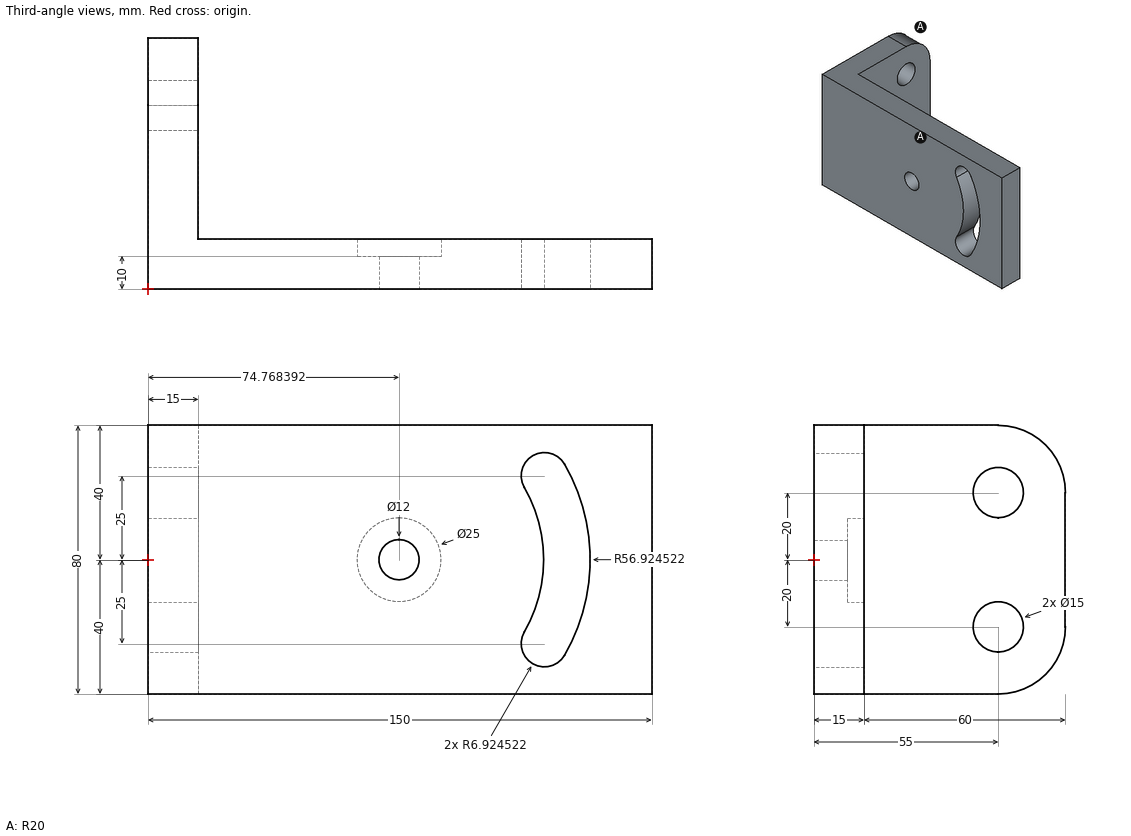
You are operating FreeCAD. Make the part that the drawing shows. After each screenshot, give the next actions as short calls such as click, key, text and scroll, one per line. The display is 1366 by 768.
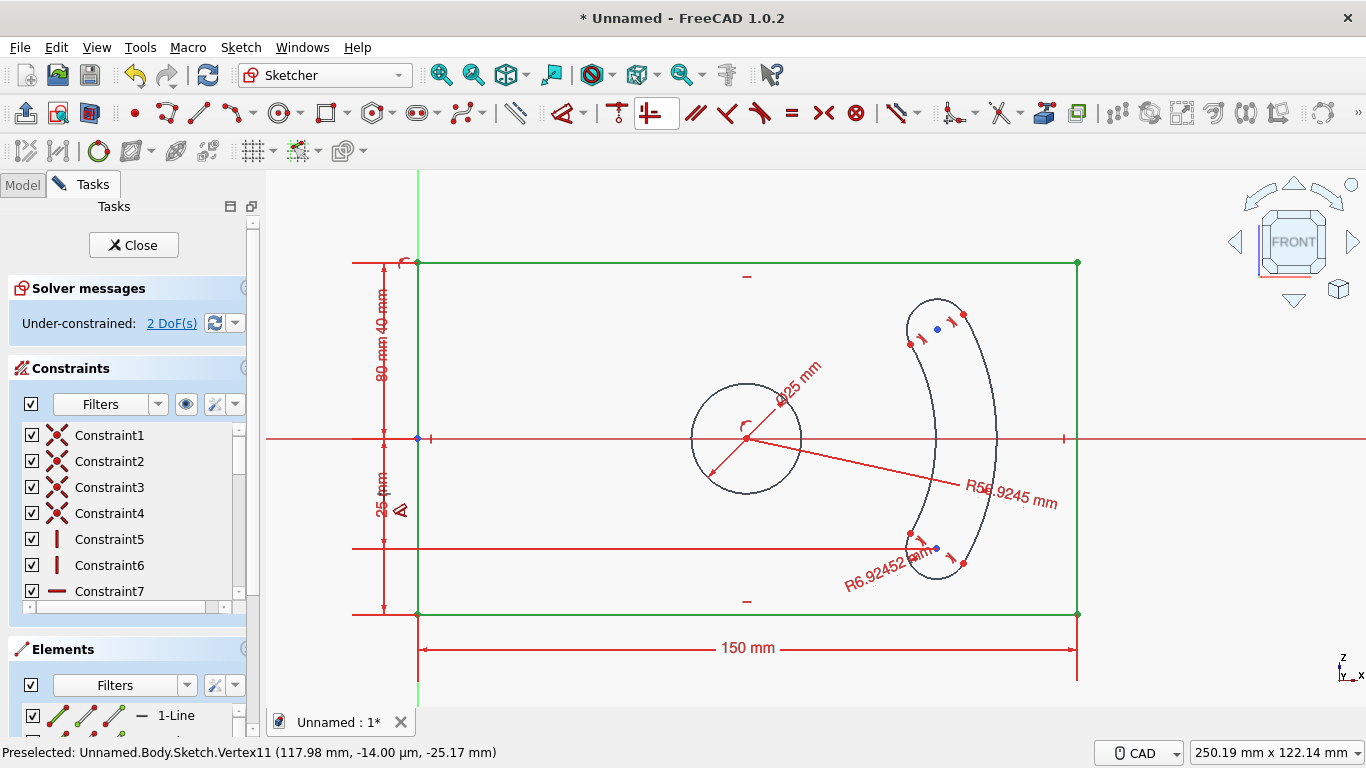
click(937, 330)
click(384, 384)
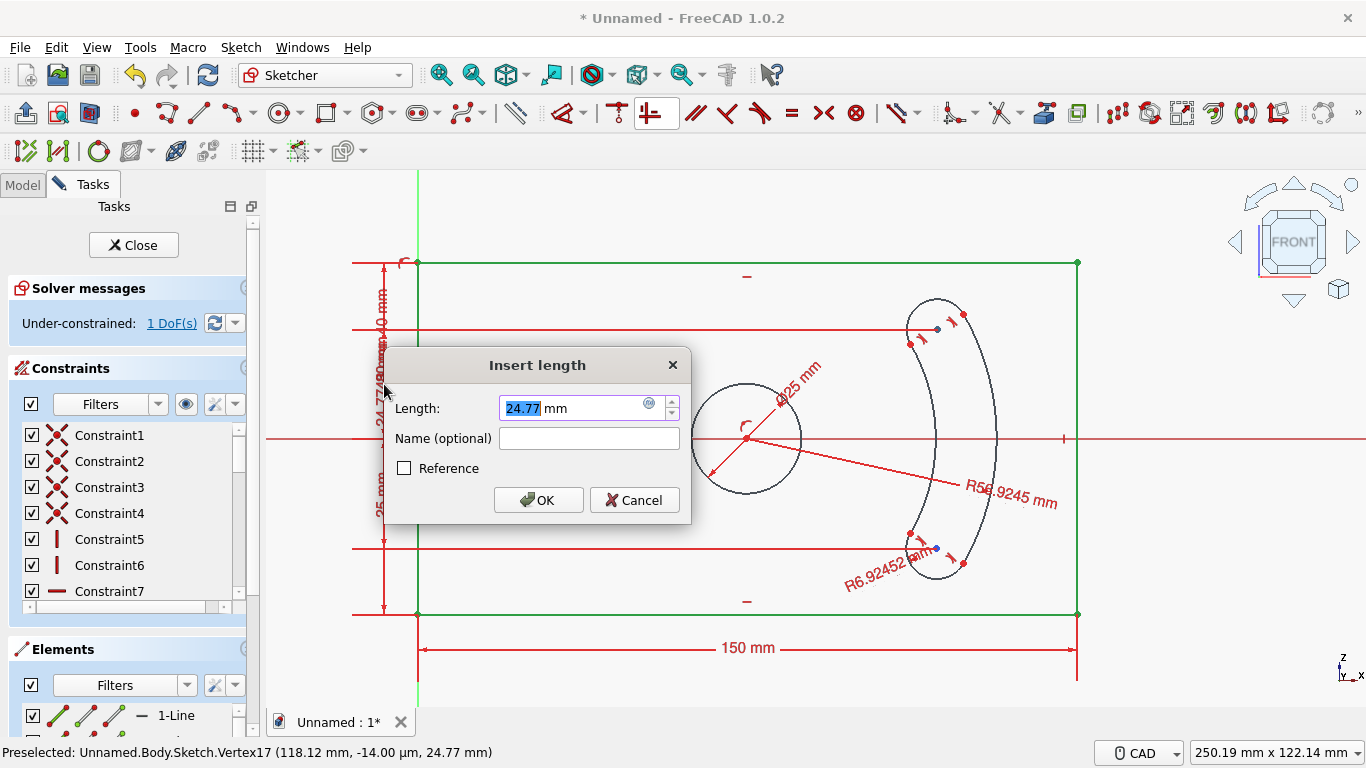
text(25)
key(Return)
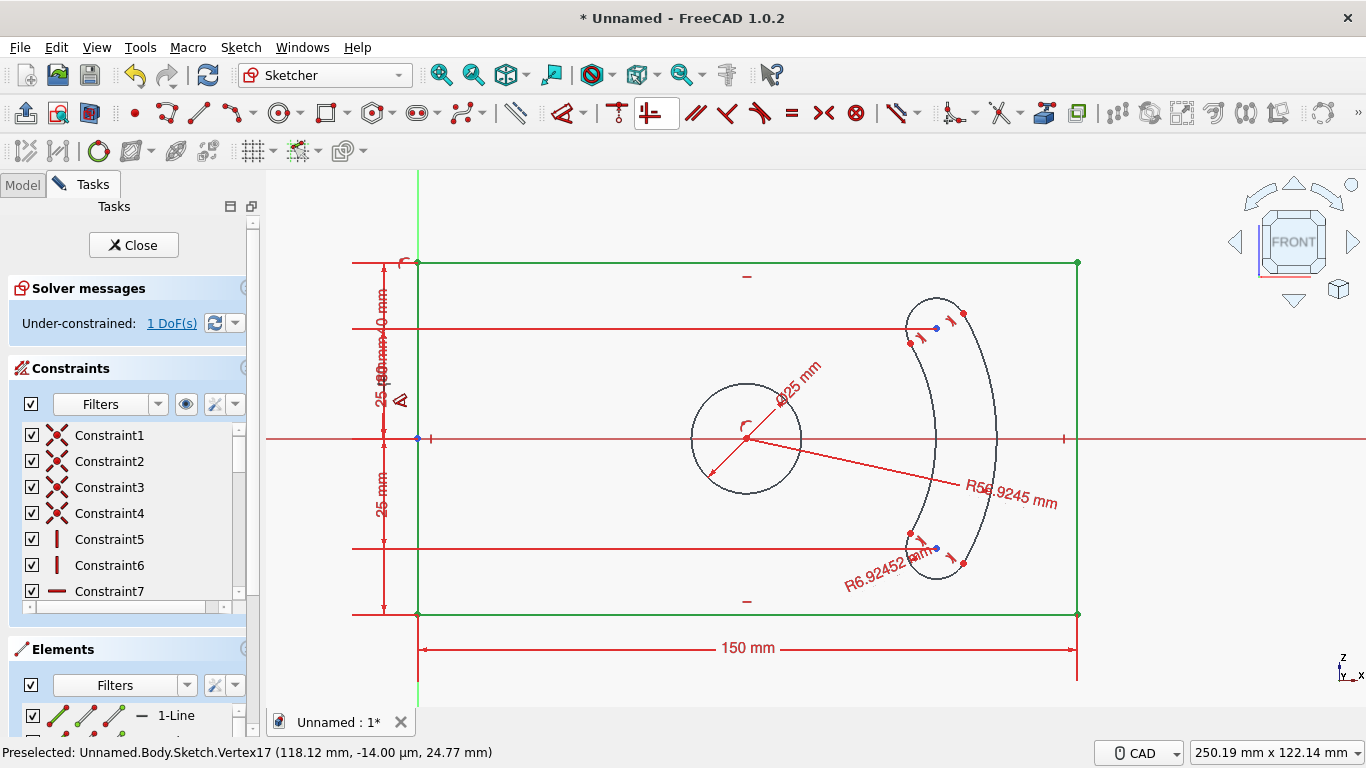
click(746, 439)
click(582, 473)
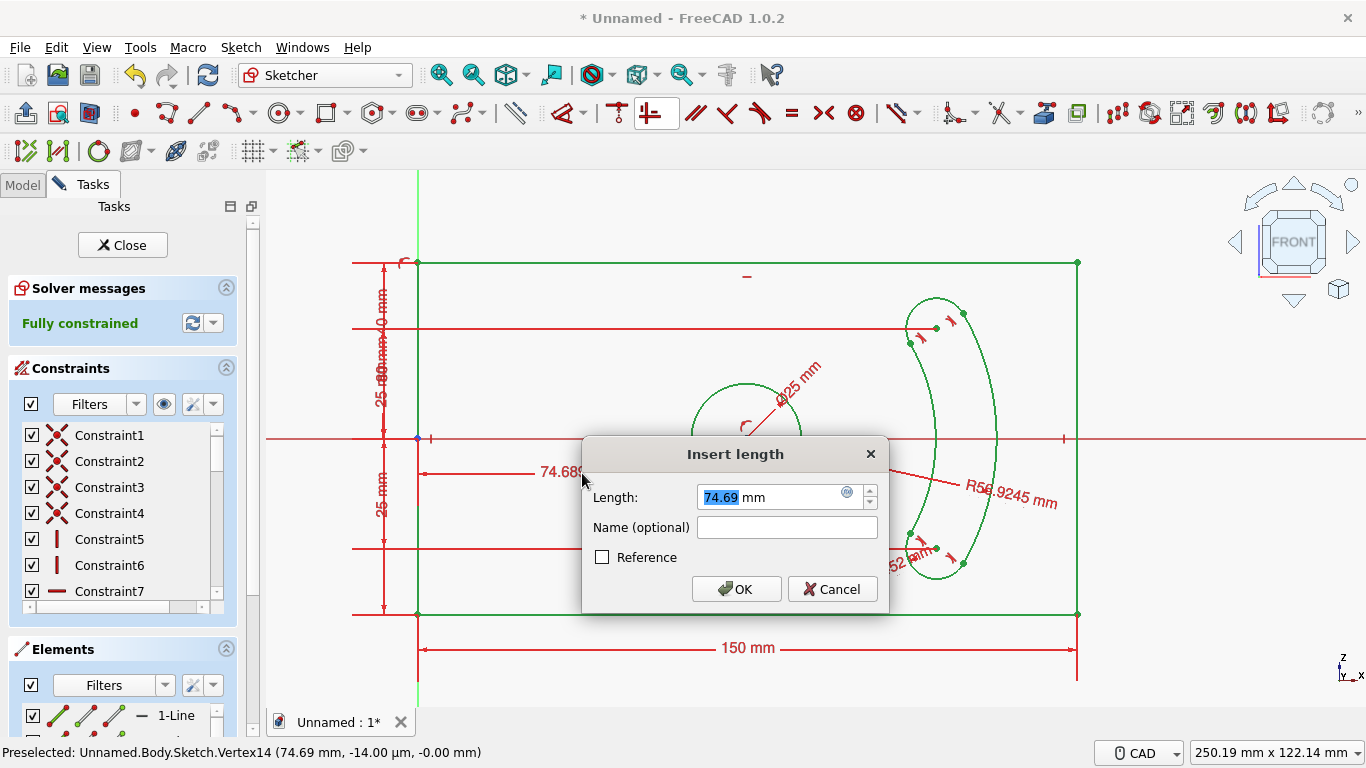
text(74.768392)
key(Return)
key(Escape)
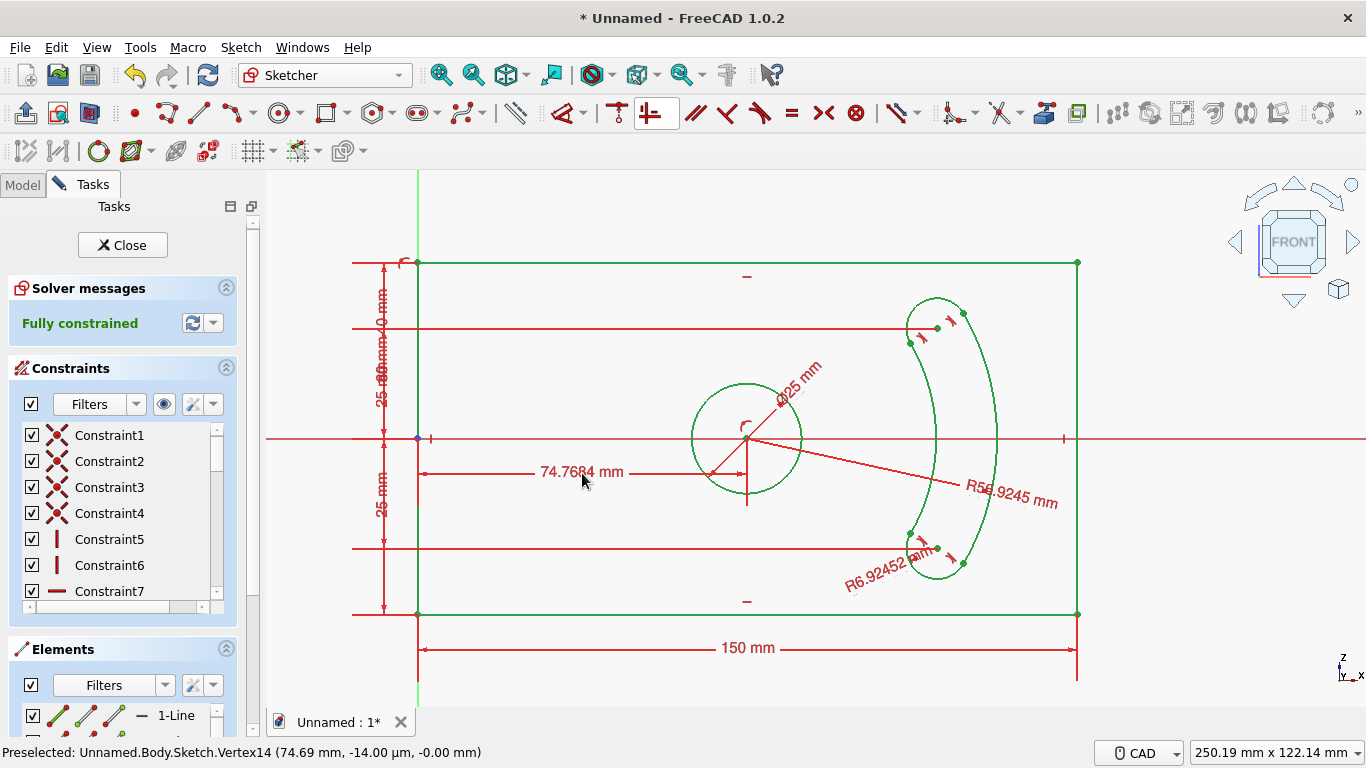
click(123, 245)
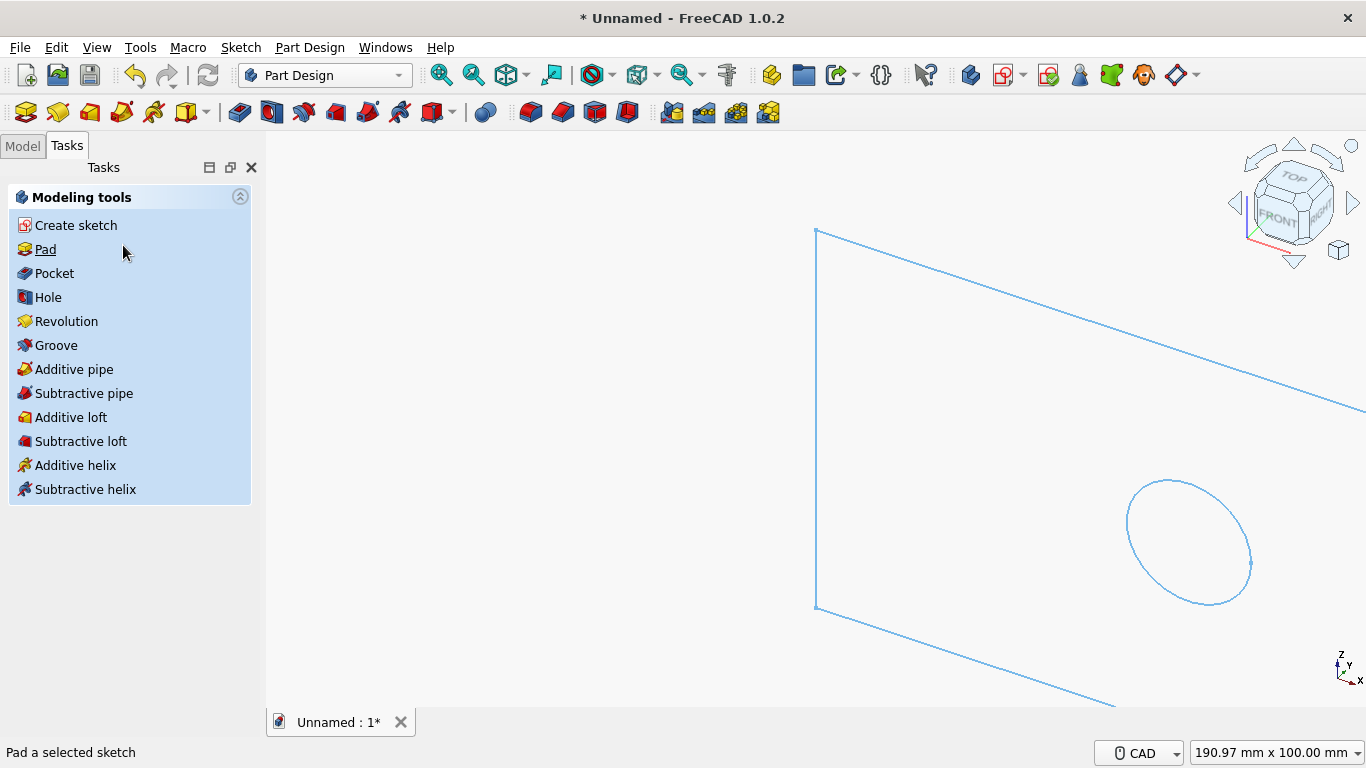
click(26, 112)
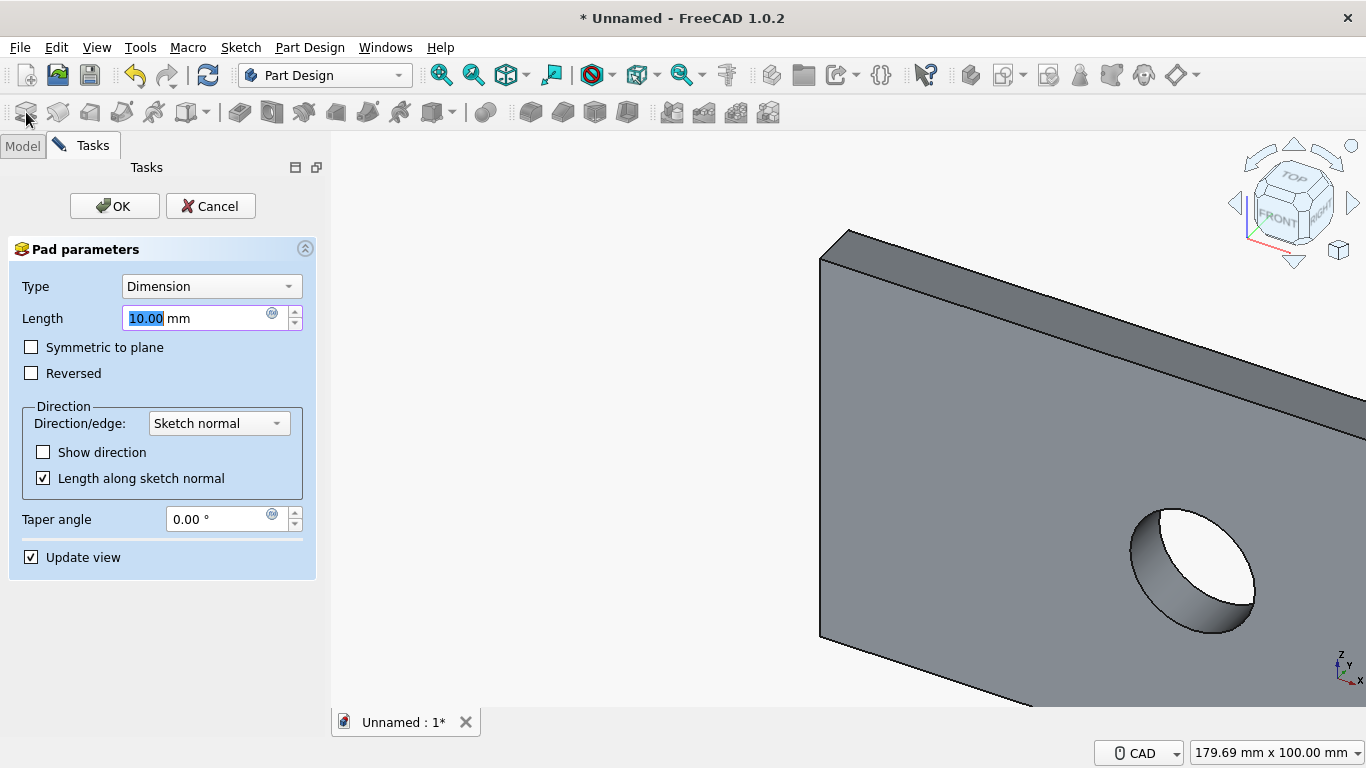
text(15)
key(Tab)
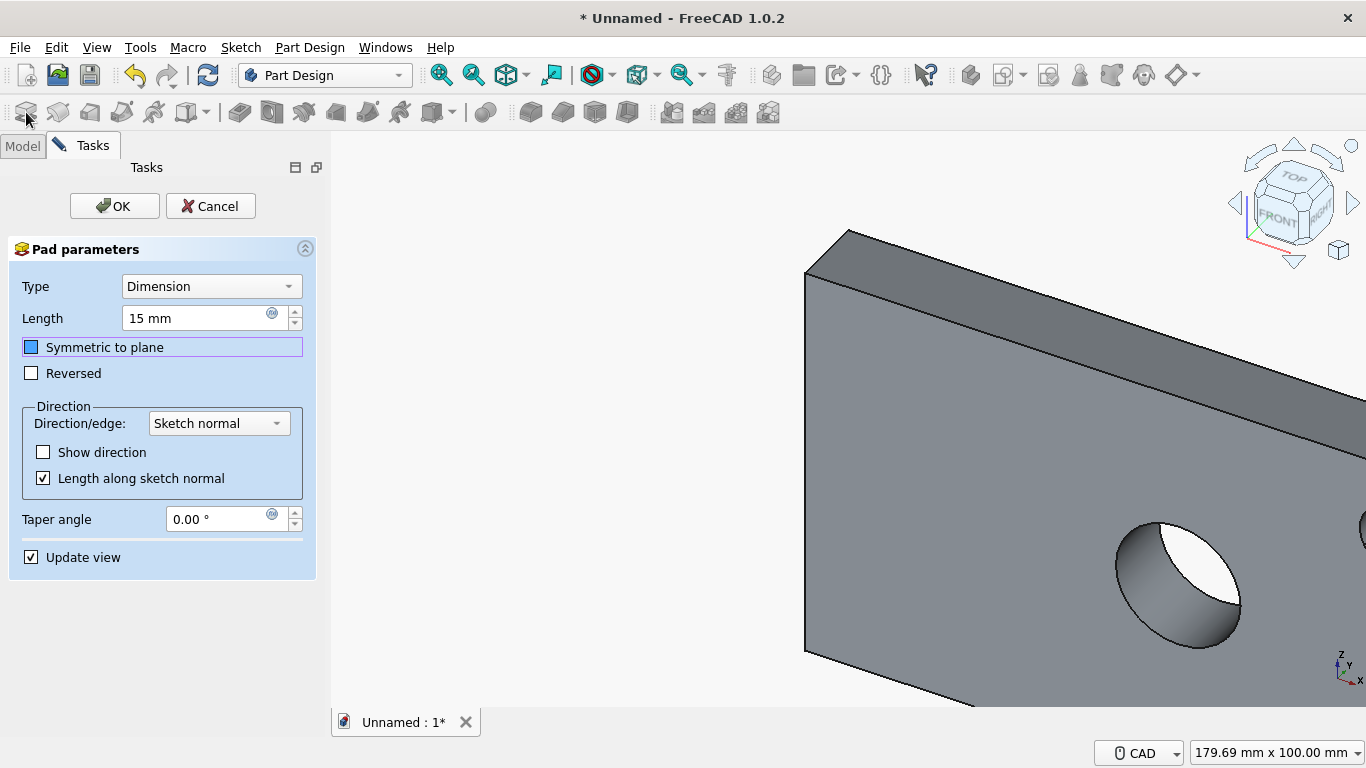
click(30, 373)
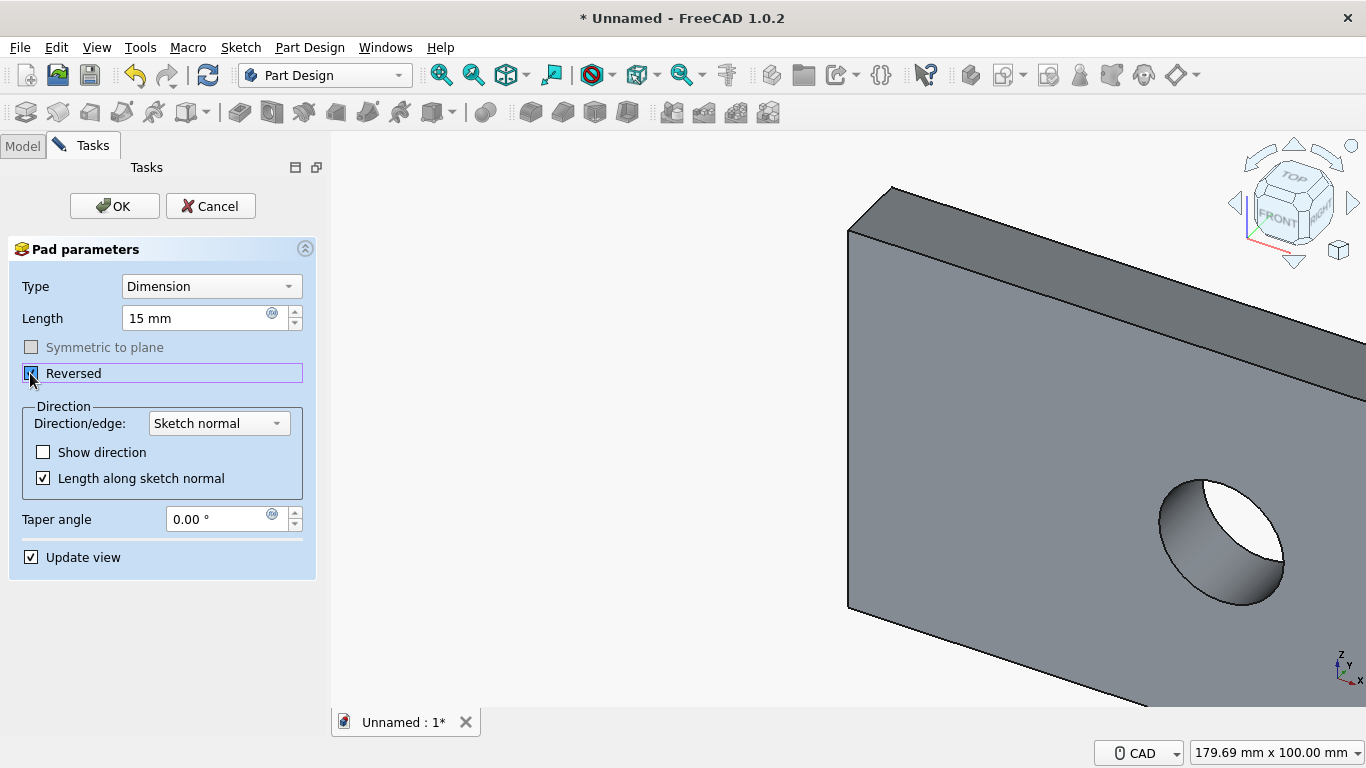
click(115, 206)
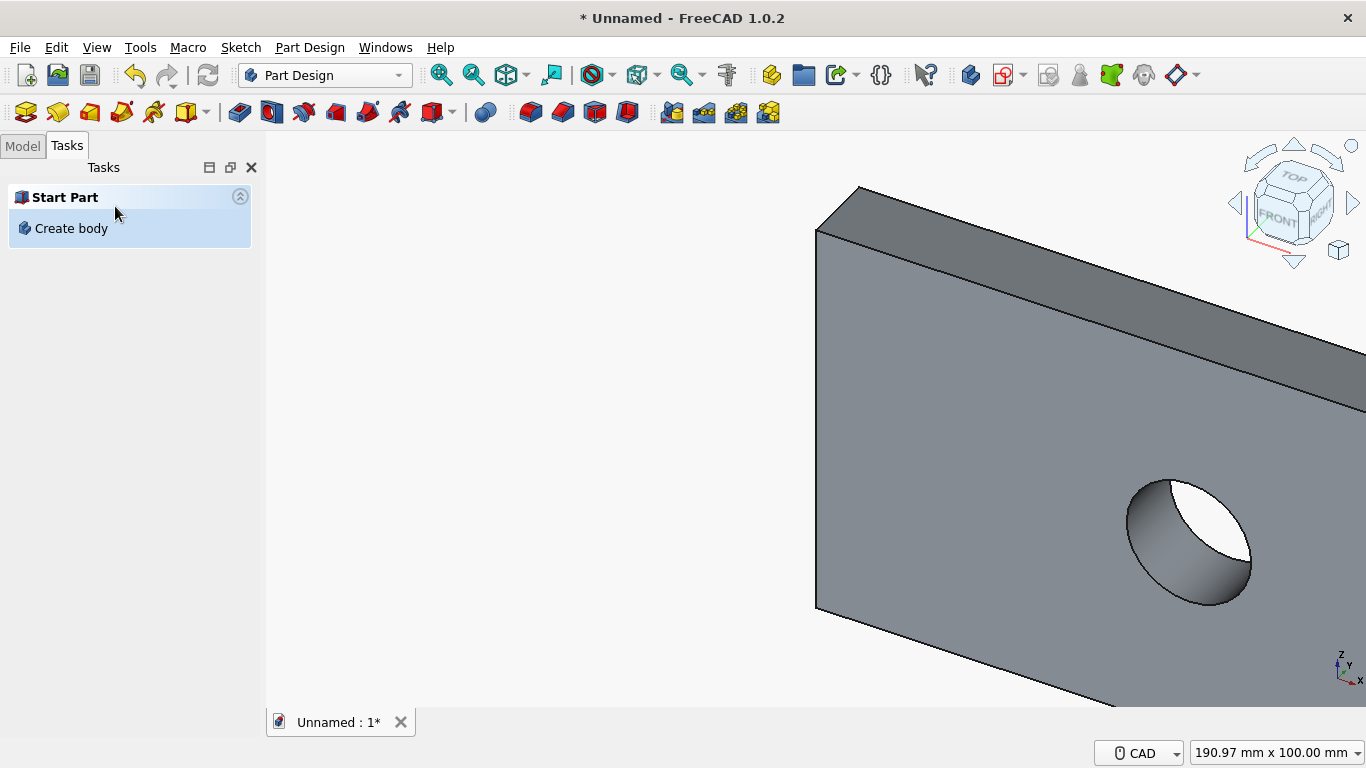
click(442, 76)